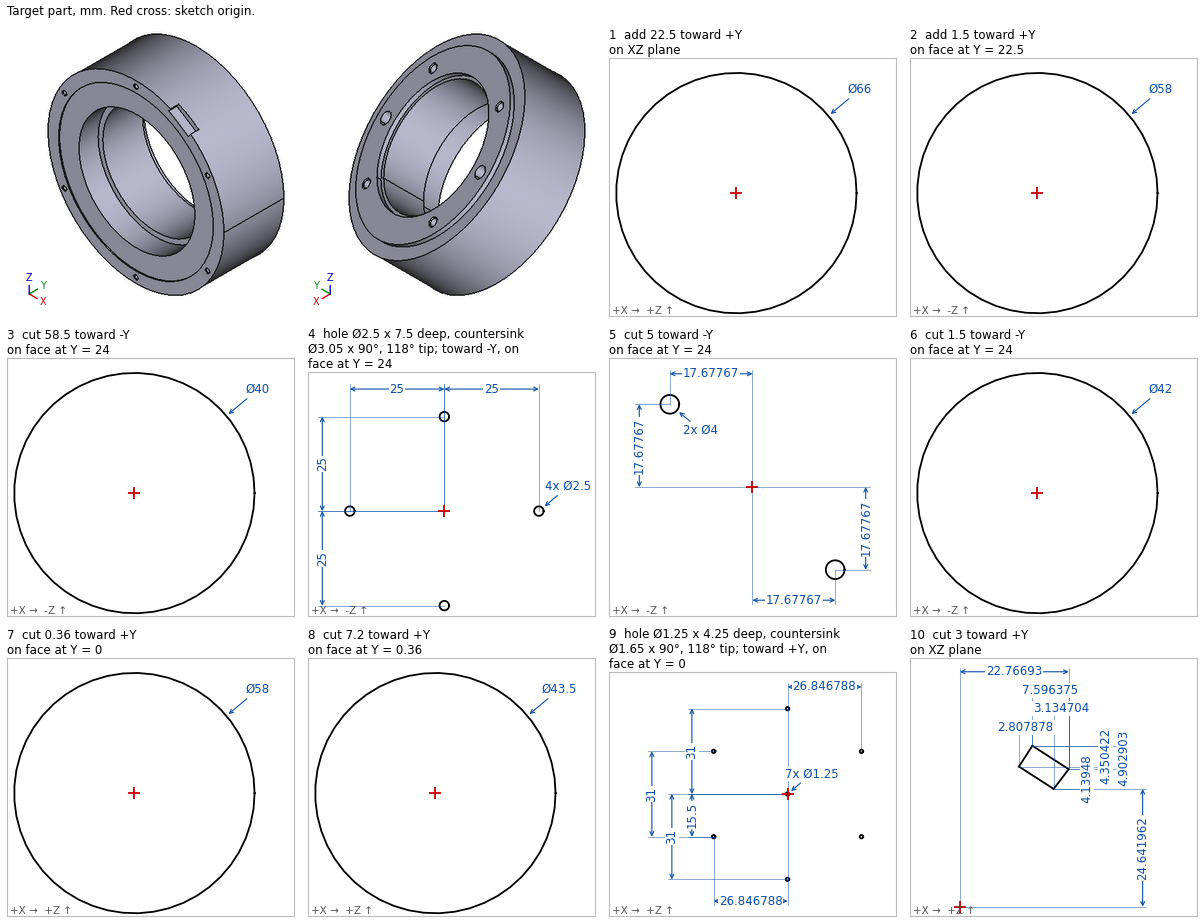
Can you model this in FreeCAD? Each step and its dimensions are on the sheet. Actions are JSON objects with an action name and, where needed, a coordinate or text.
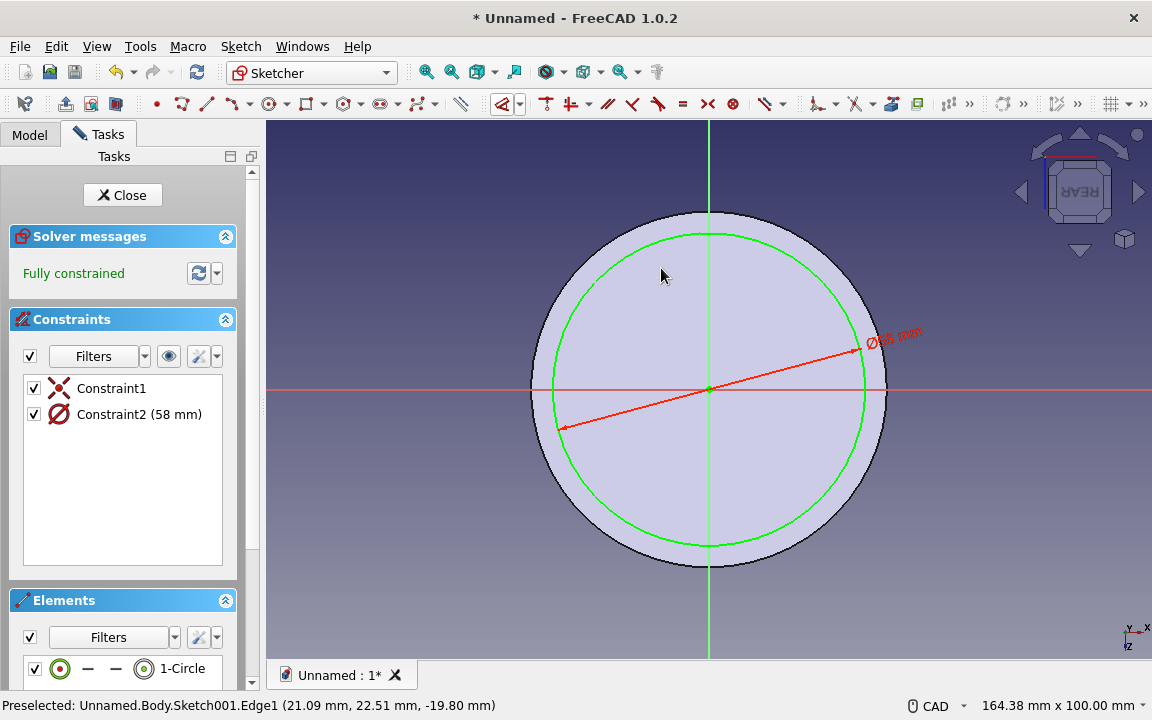
{"action": "left_click", "coordinate": [123, 195]}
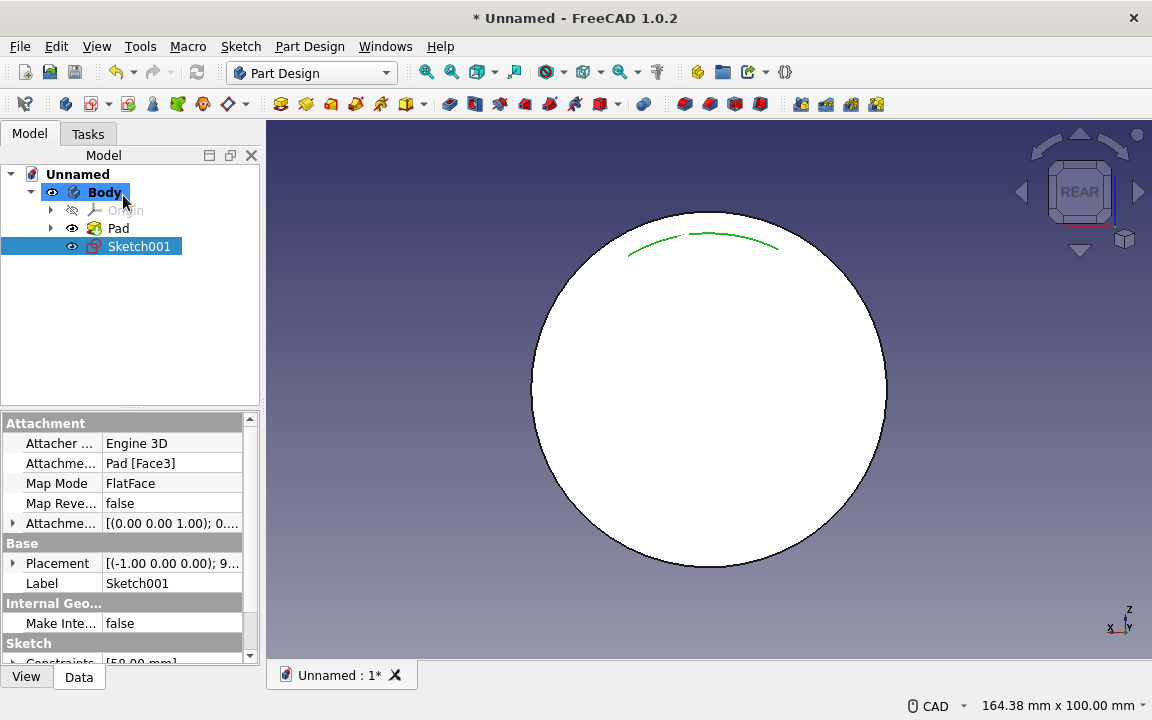
{"action": "left_click", "coordinate": [281, 104]}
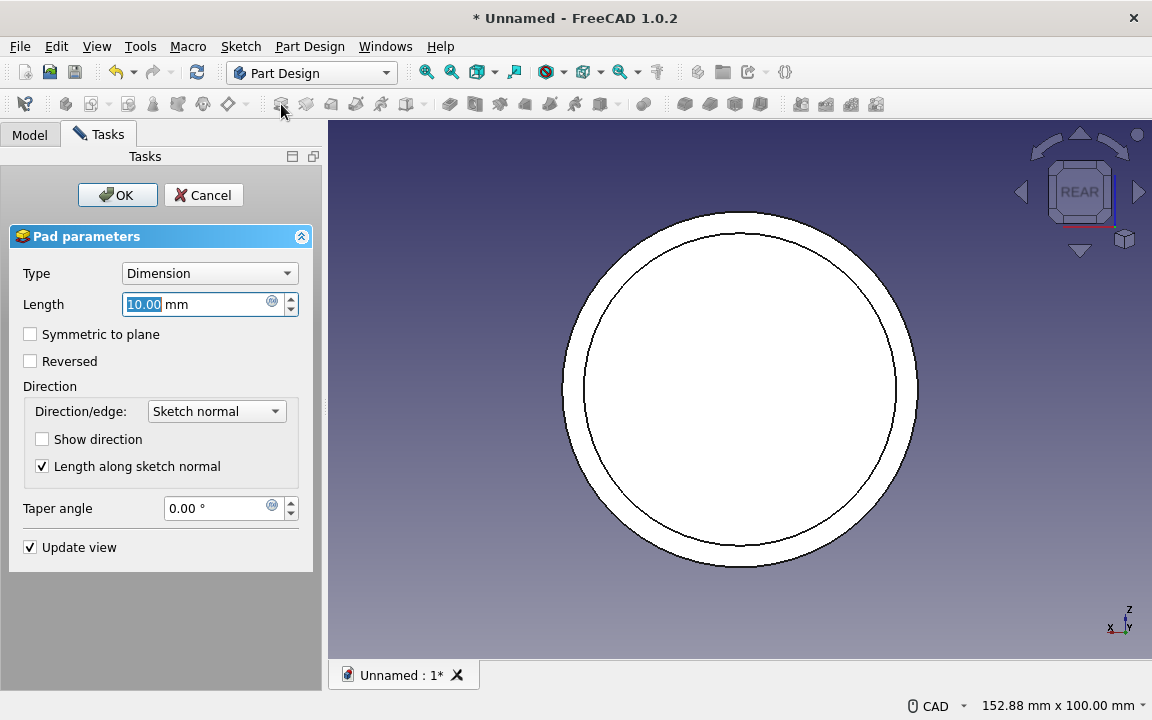
{"action": "type", "text": "1.5"}
{"action": "key", "text": "Tab"}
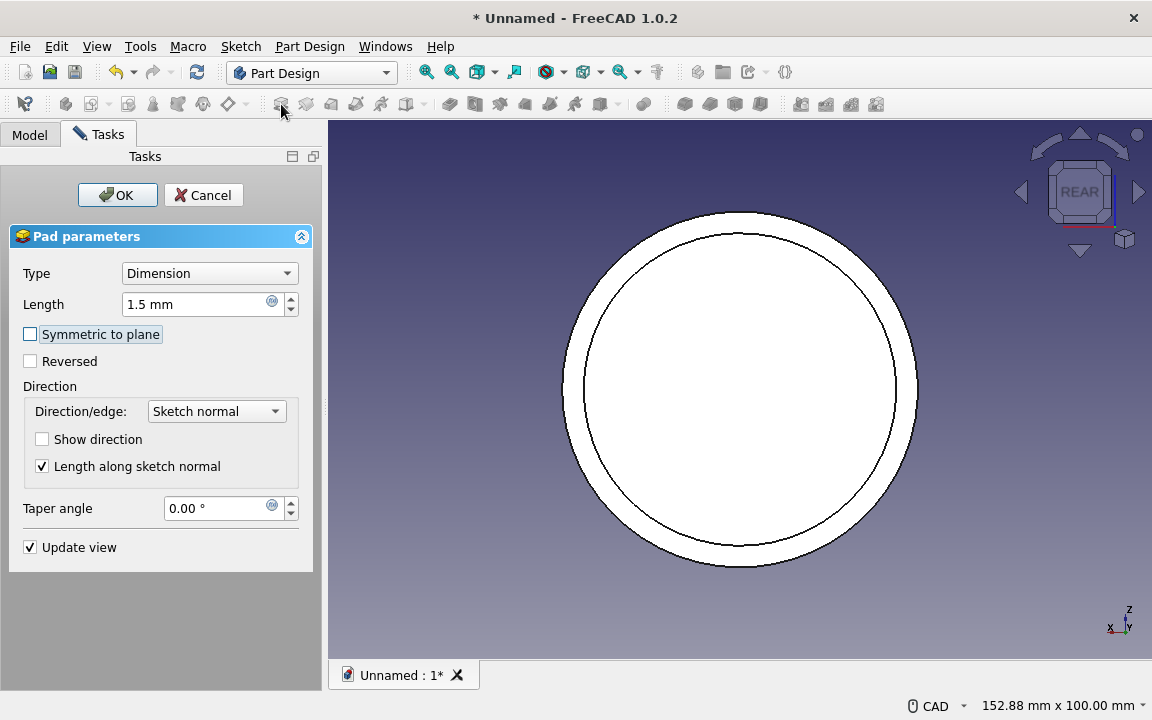
{"action": "left_click", "coordinate": [118, 195]}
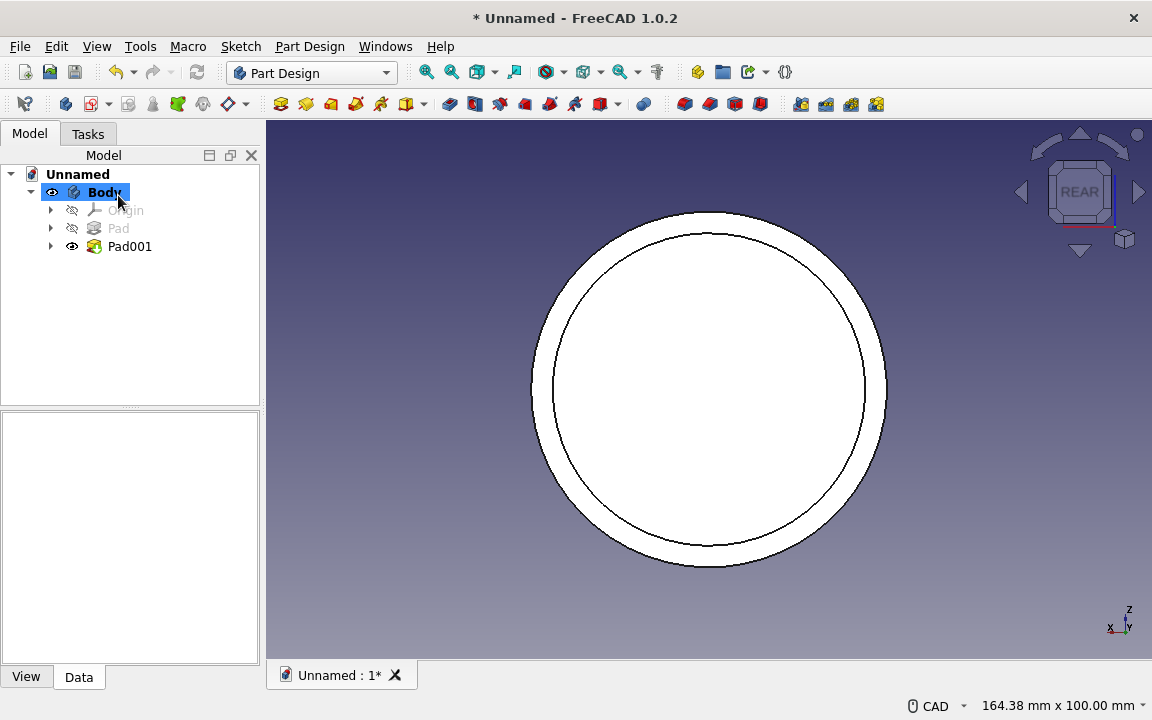
{"action": "left_click", "coordinate": [709, 388]}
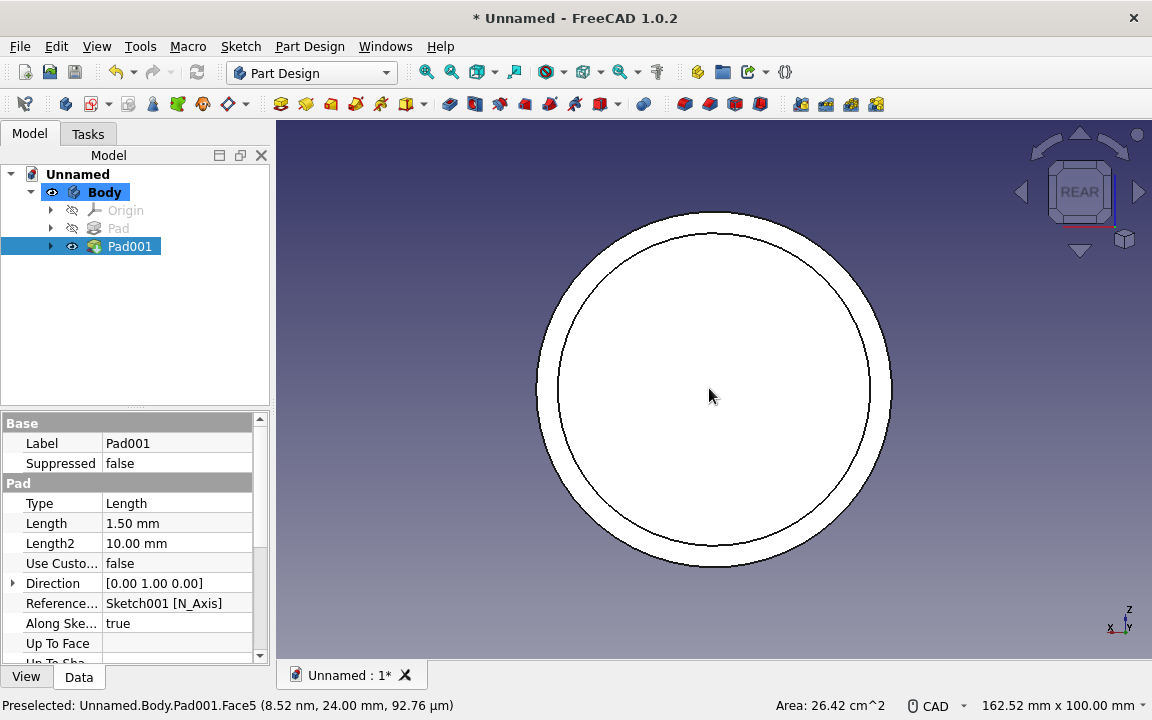
{"action": "left_click", "coordinate": [90, 104]}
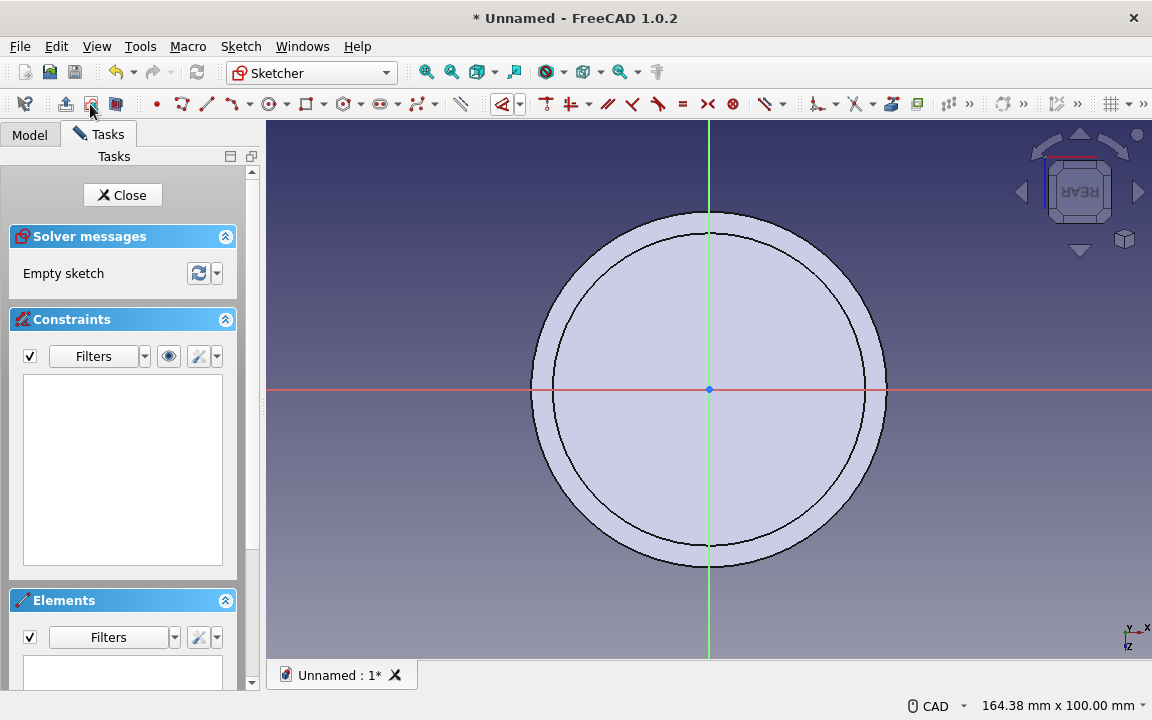
{"action": "scroll", "coordinate": [848, 389], "scroll_direction": "up", "scroll_amount": 2}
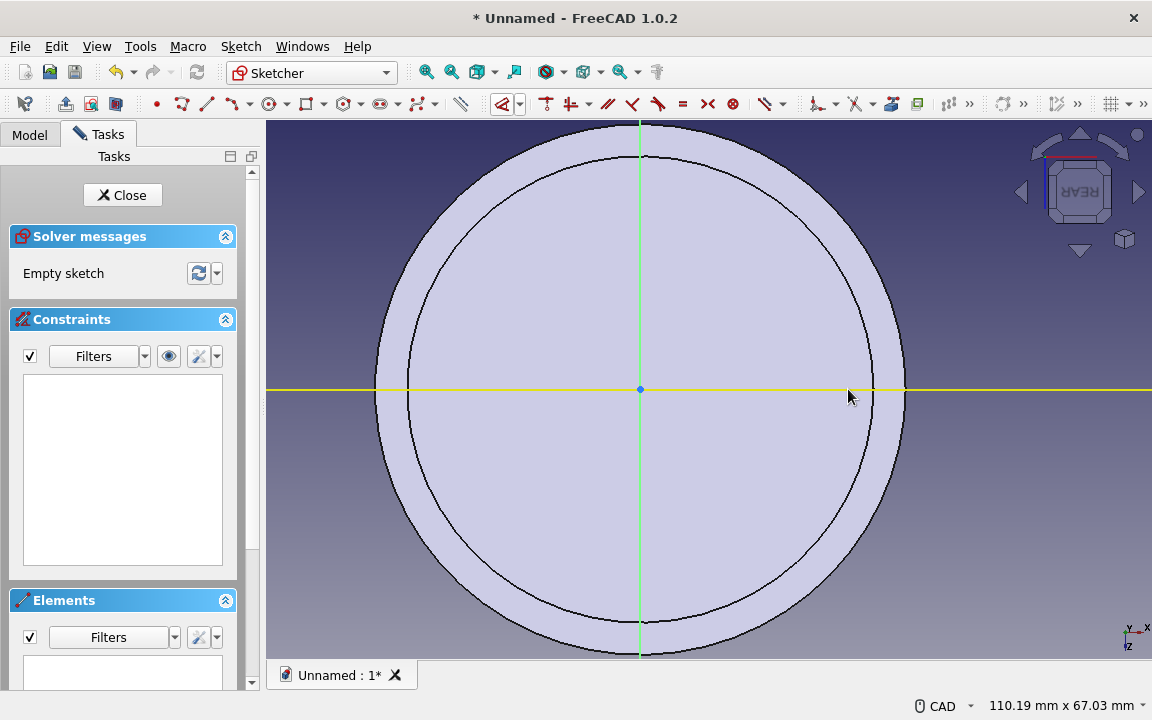
{"action": "left_click", "coordinate": [268, 104]}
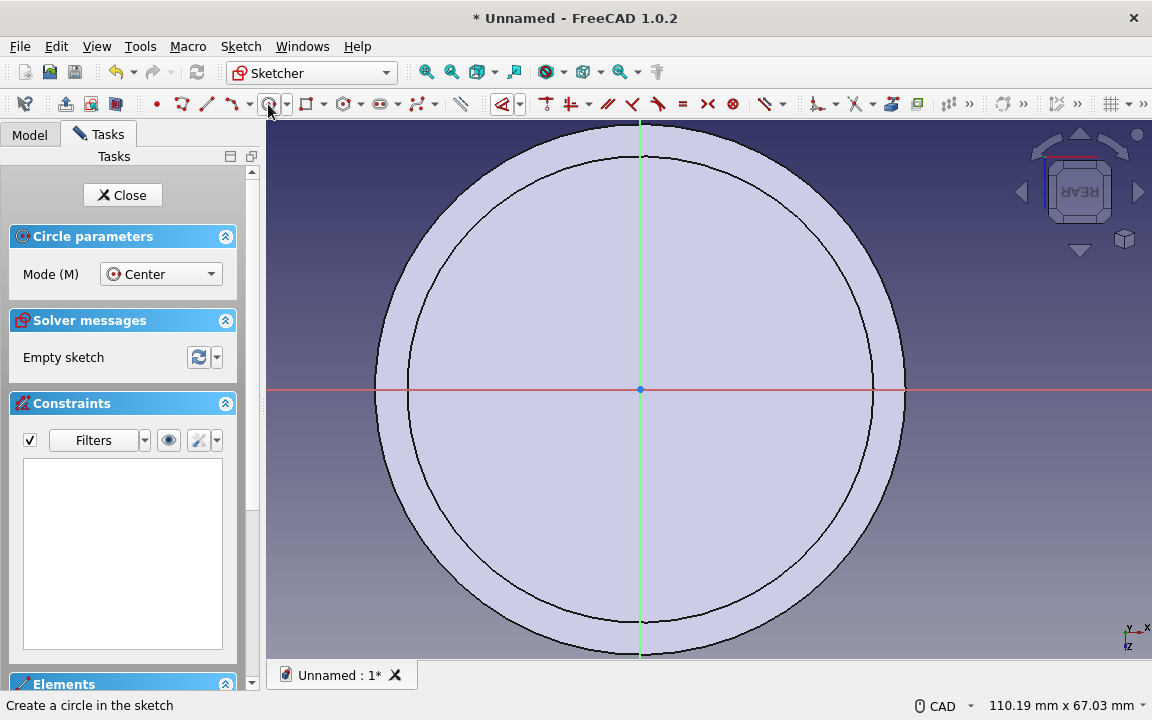
{"action": "left_click", "coordinate": [640, 389]}
{"action": "left_click", "coordinate": [754, 276]}
{"action": "key", "text": "Escape"}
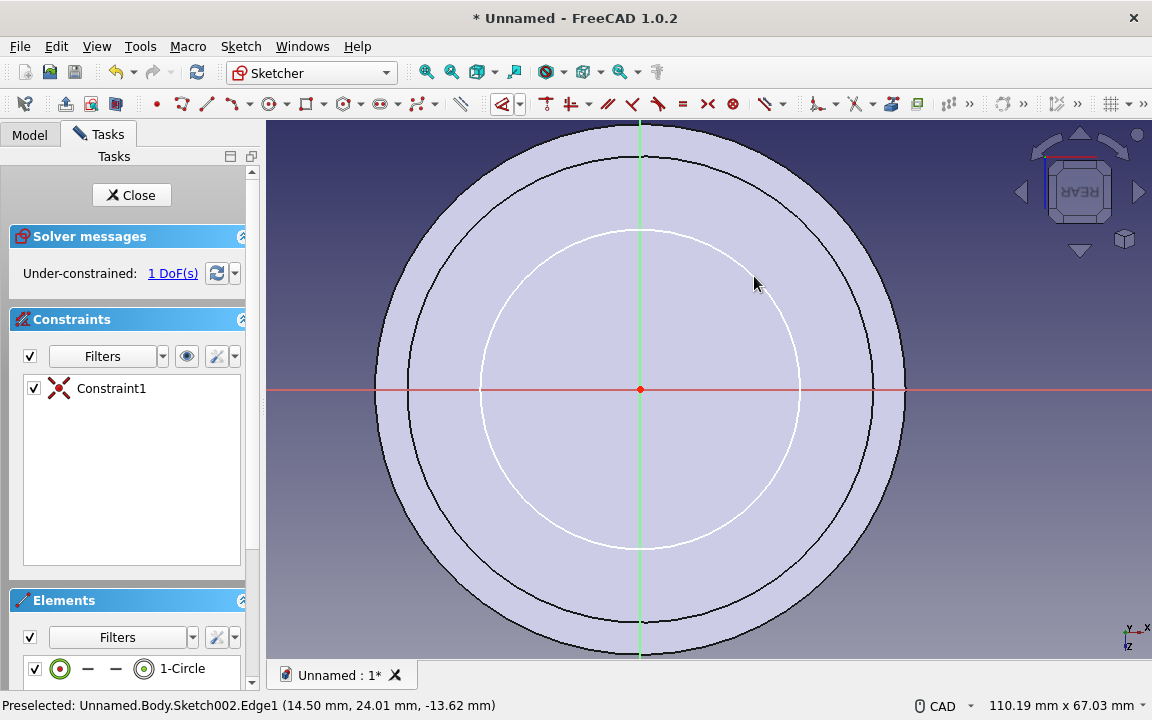
{"action": "left_click", "coordinate": [753, 276]}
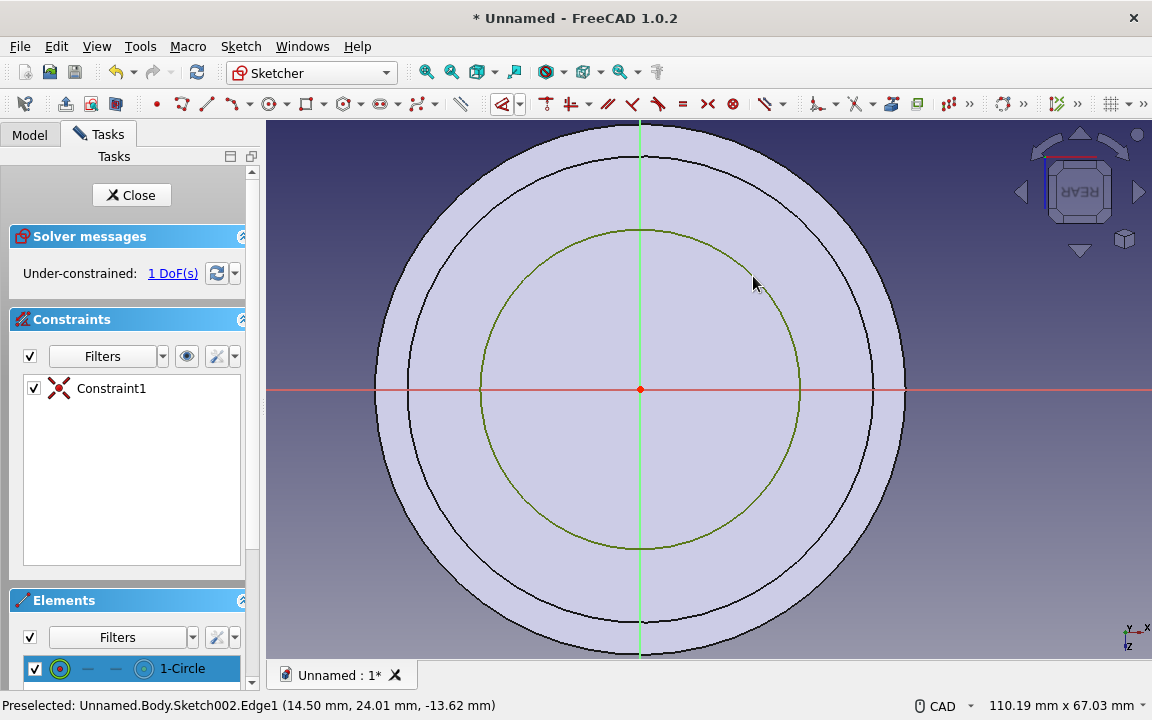
{"action": "left_click", "coordinate": [520, 104]}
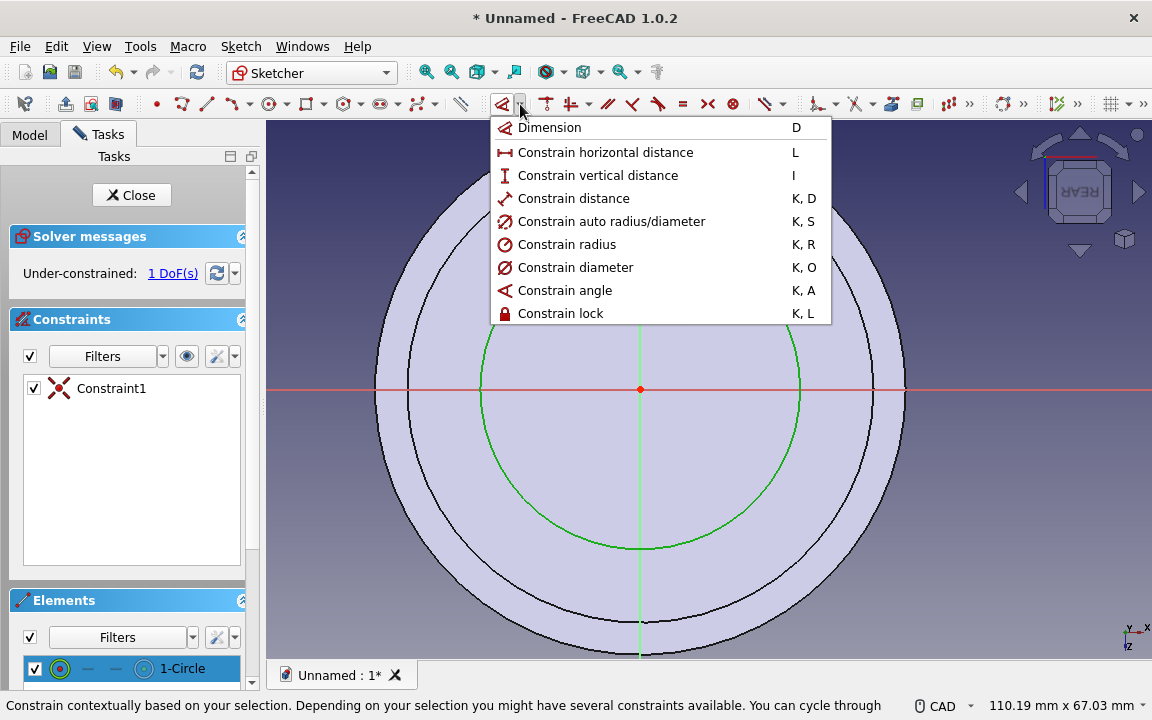
{"action": "left_click", "coordinate": [661, 268]}